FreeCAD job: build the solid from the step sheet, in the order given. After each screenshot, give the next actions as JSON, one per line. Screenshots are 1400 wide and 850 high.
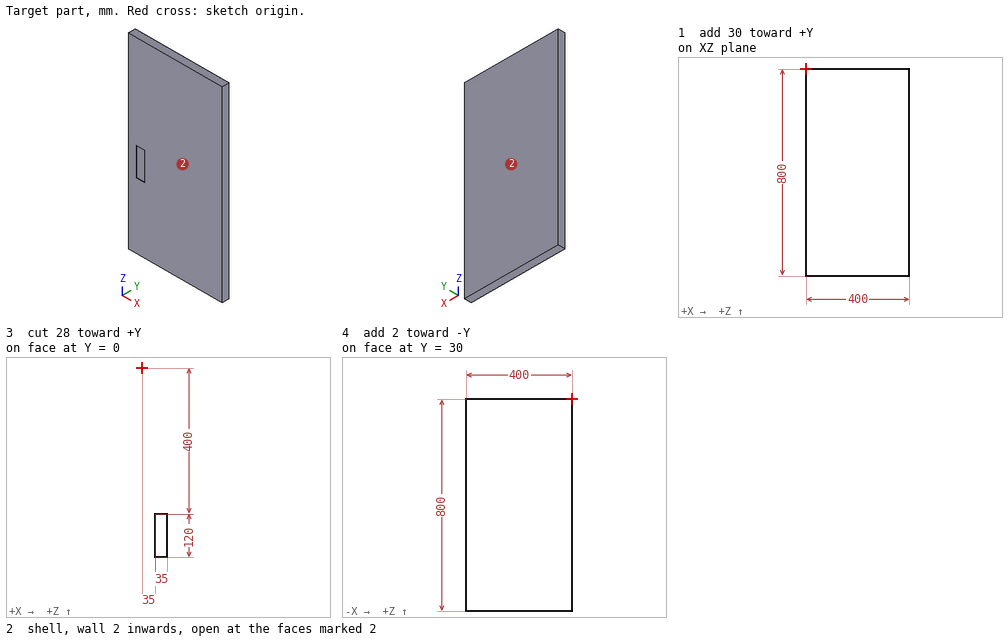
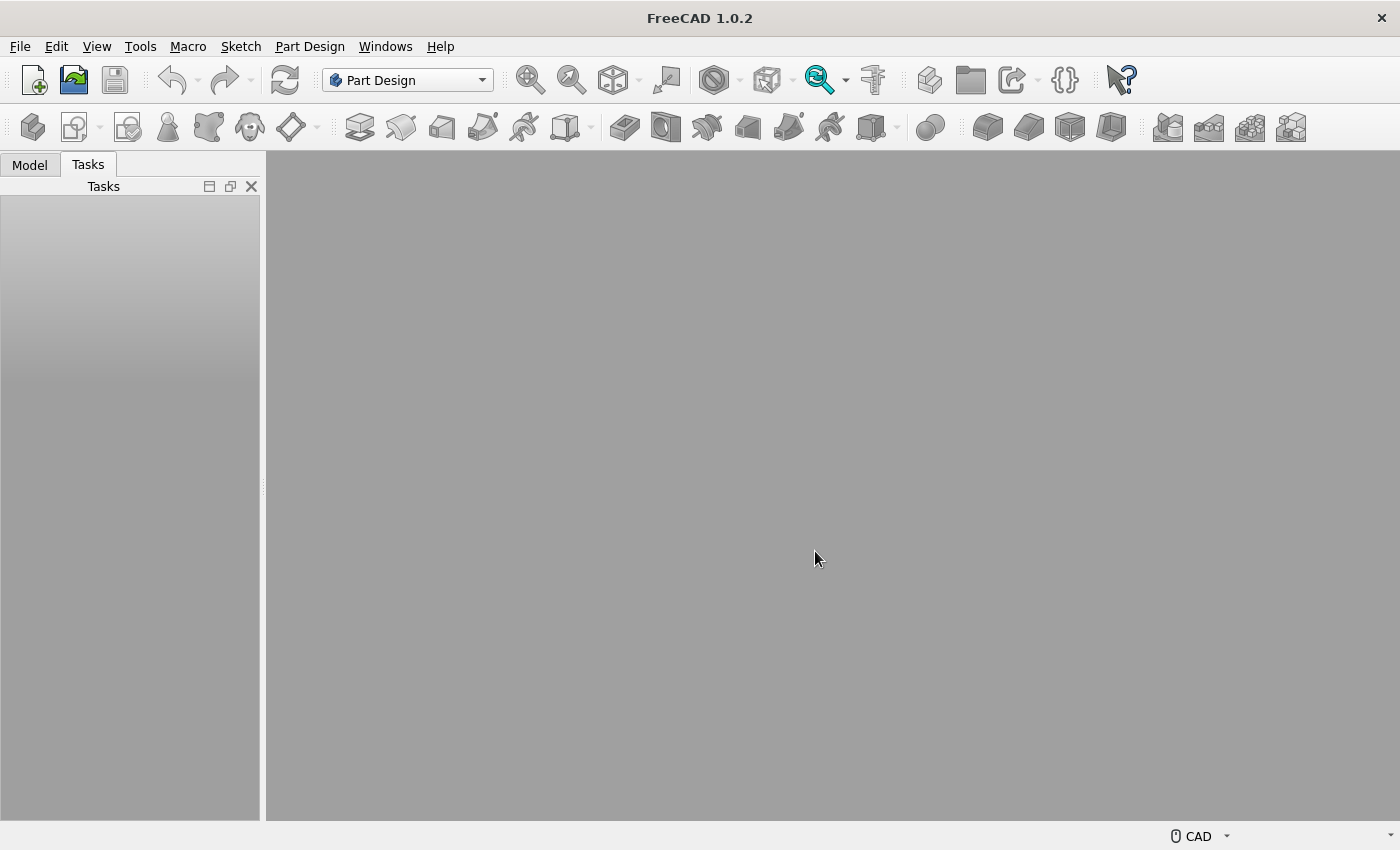
{"action": "left_click", "coordinate": [33, 80]}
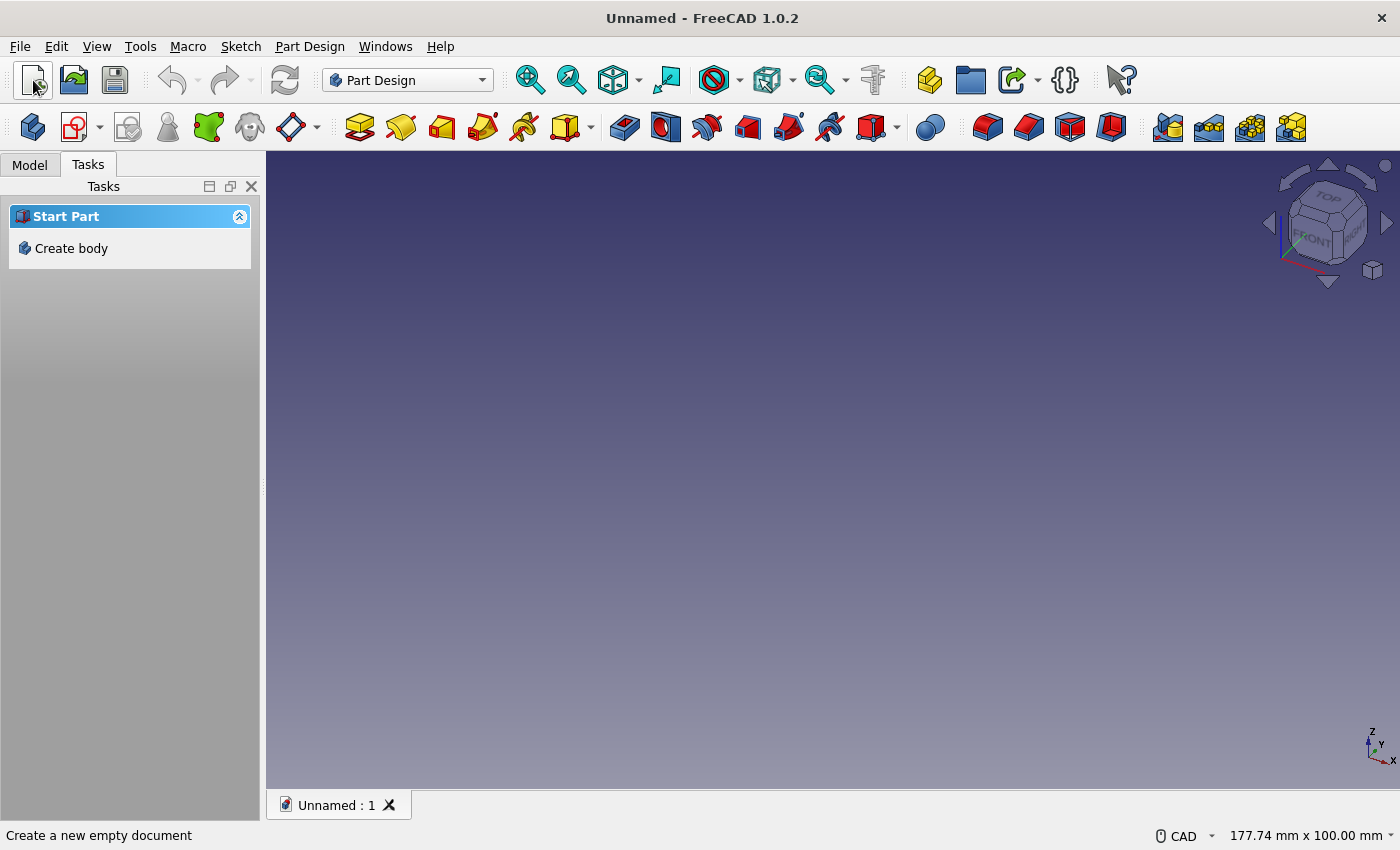
{"action": "left_click", "coordinate": [74, 128]}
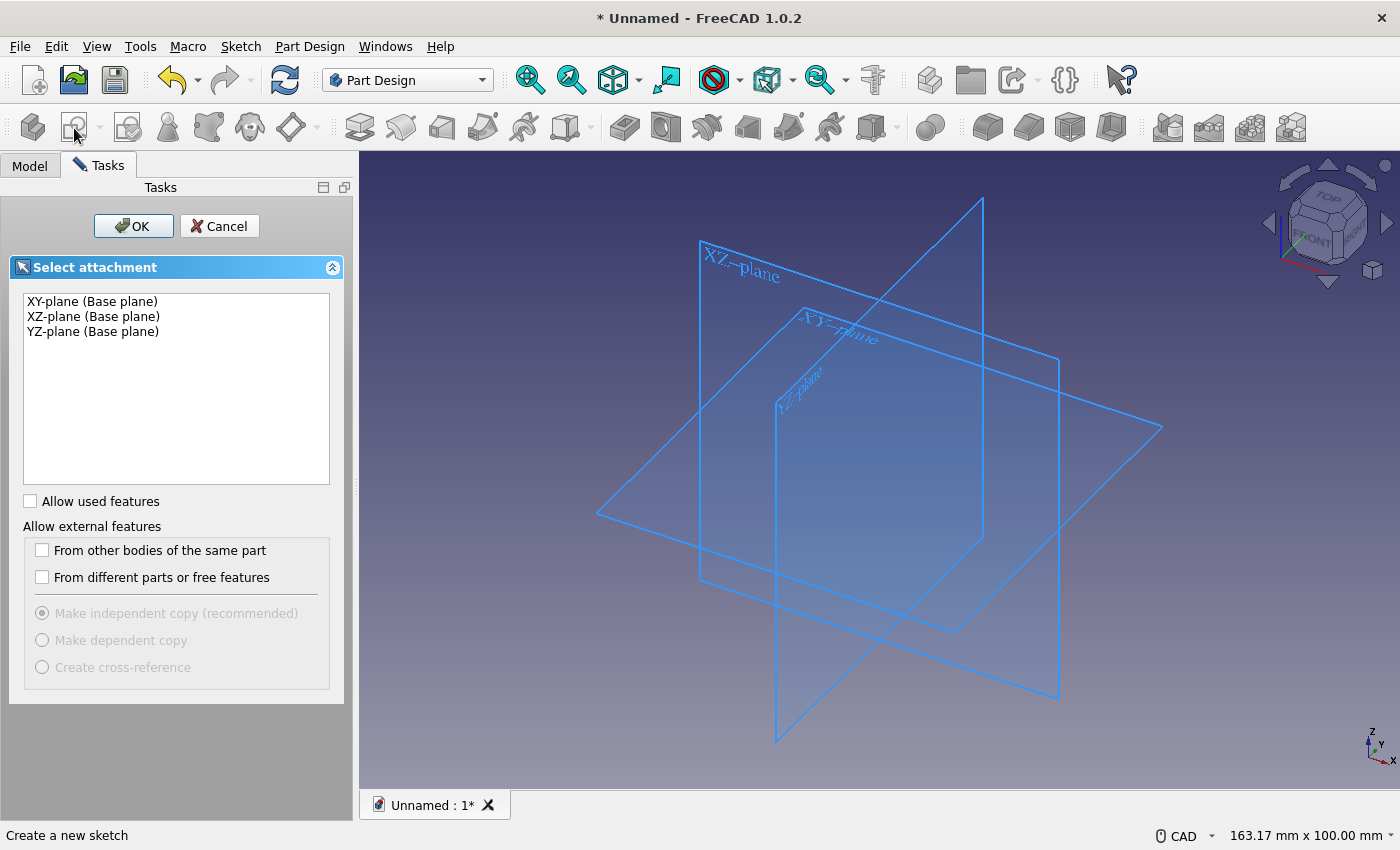
{"action": "left_click", "coordinate": [84, 316]}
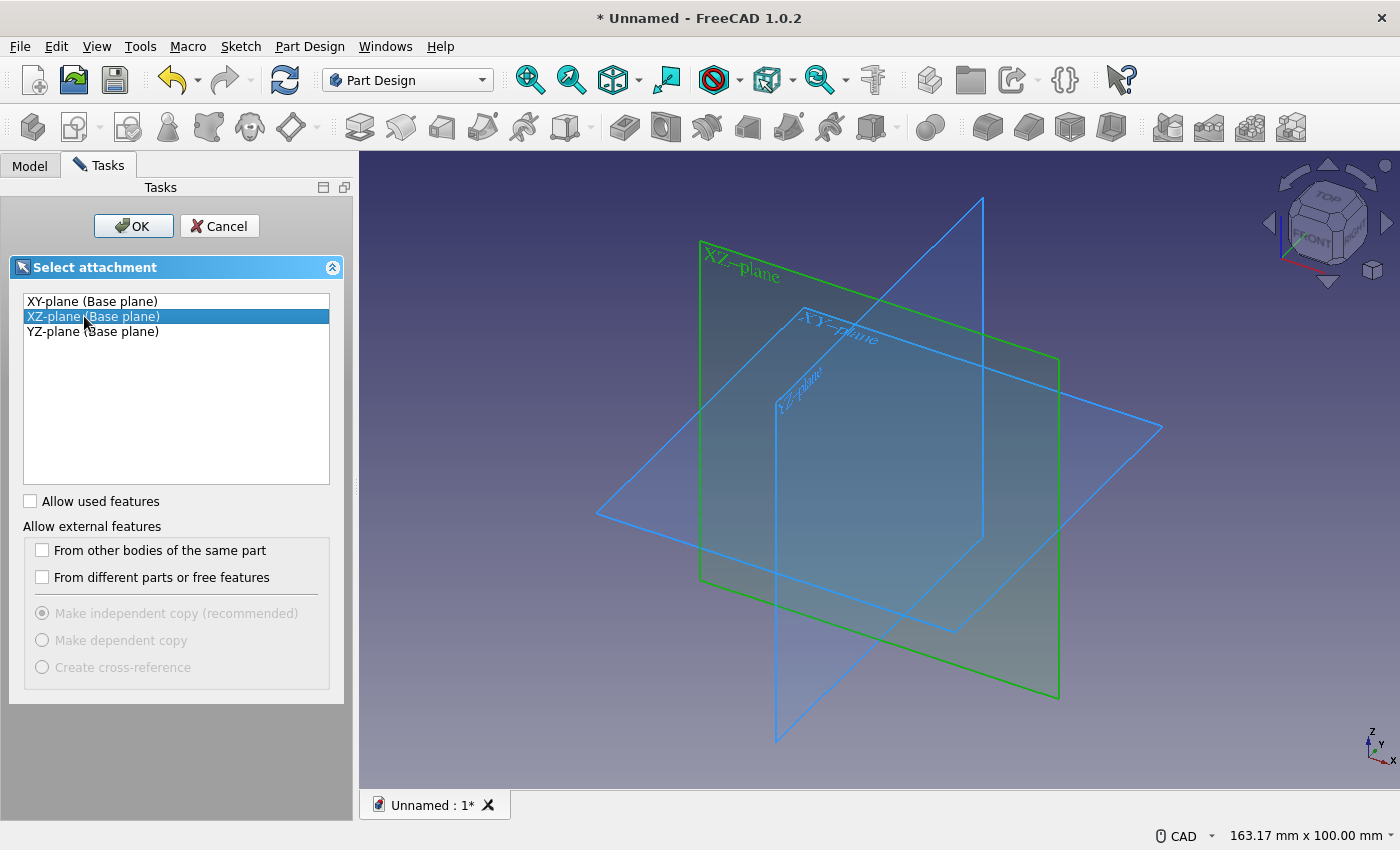
{"action": "left_click", "coordinate": [134, 226]}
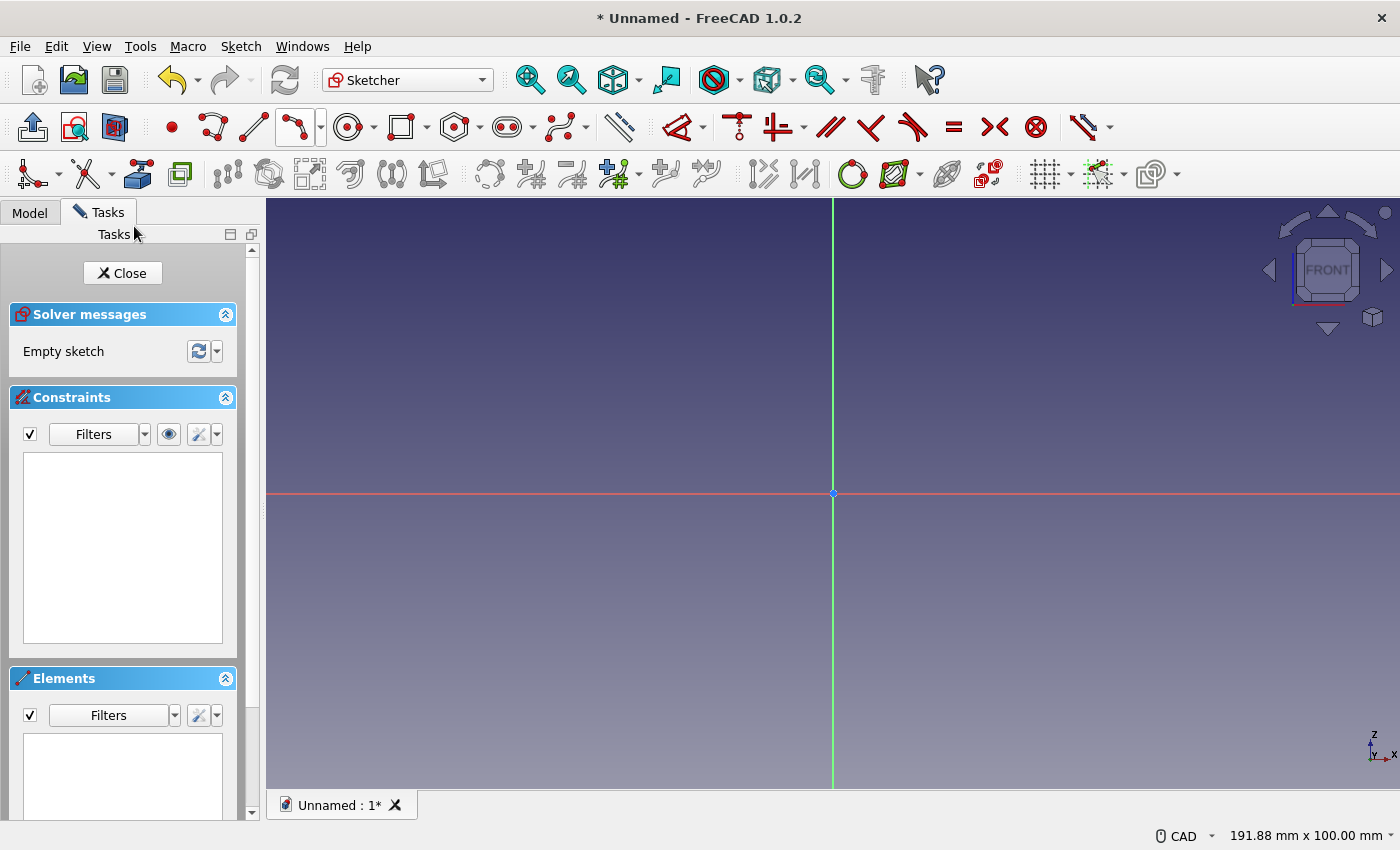
{"action": "scroll", "coordinate": [664, 304], "scroll_direction": "down", "scroll_amount": 13}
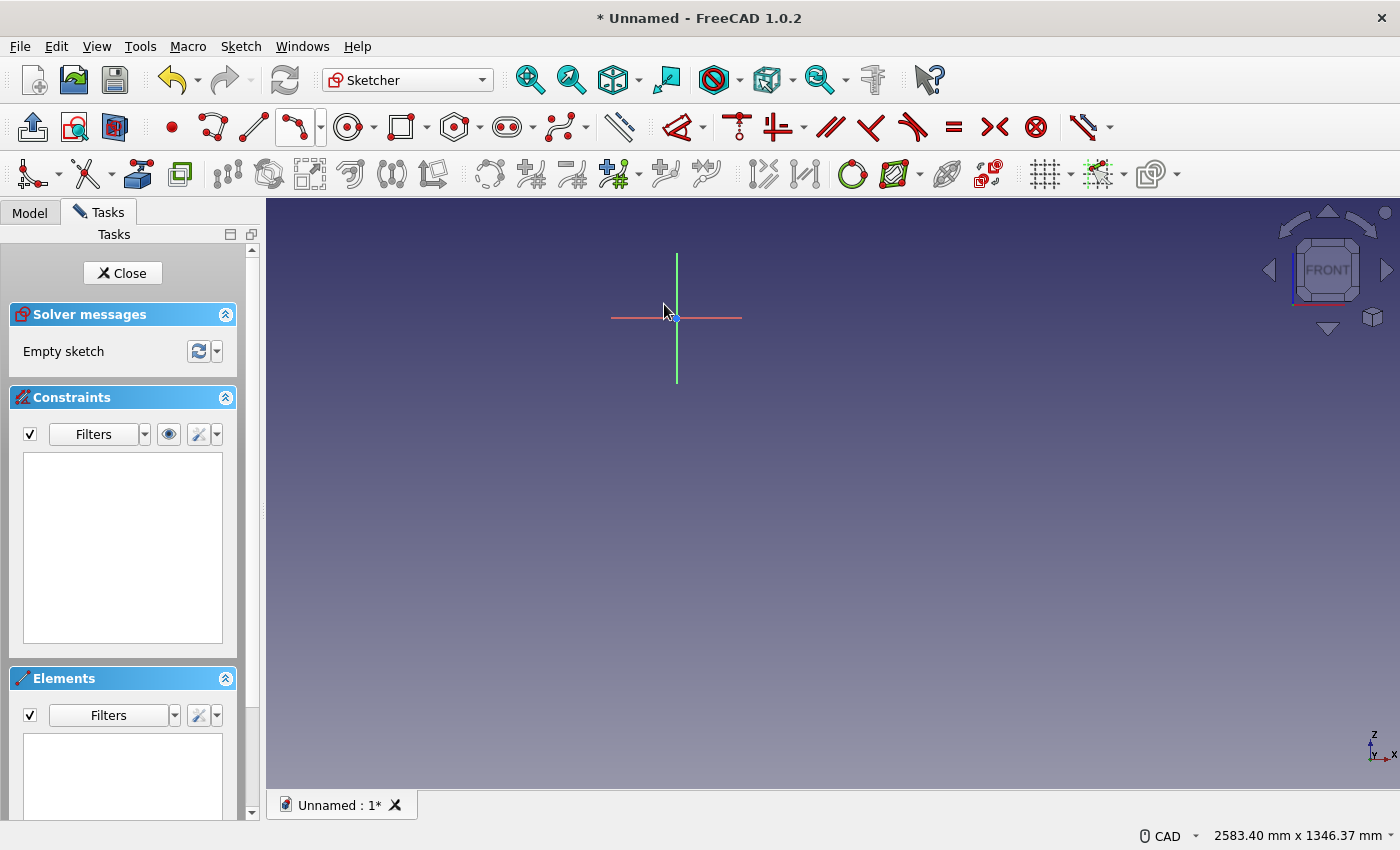
{"action": "key", "text": "g r"}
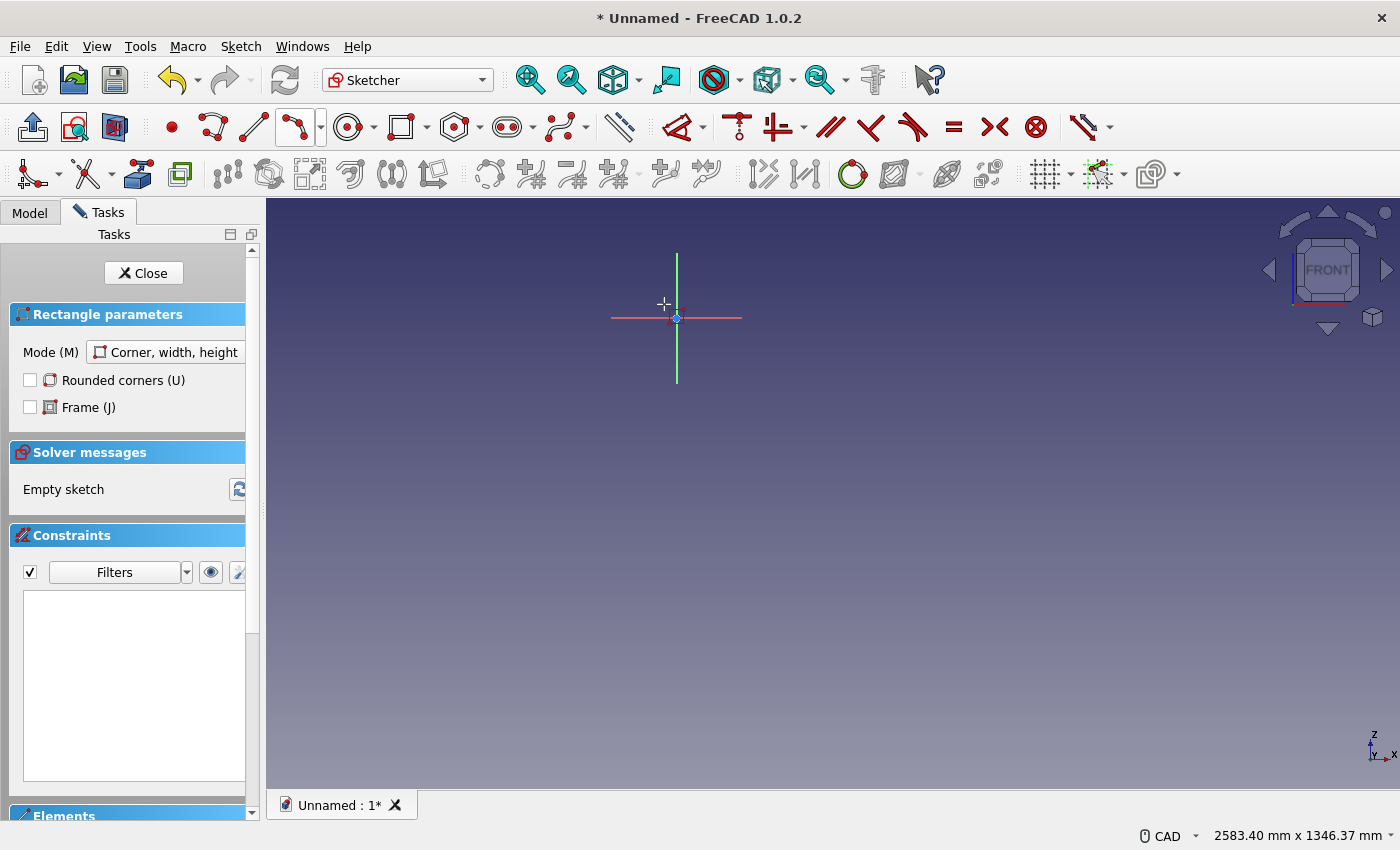
{"action": "left_click", "coordinate": [677, 318]}
{"action": "left_click", "coordinate": [852, 669]}
{"action": "key", "text": "Escape"}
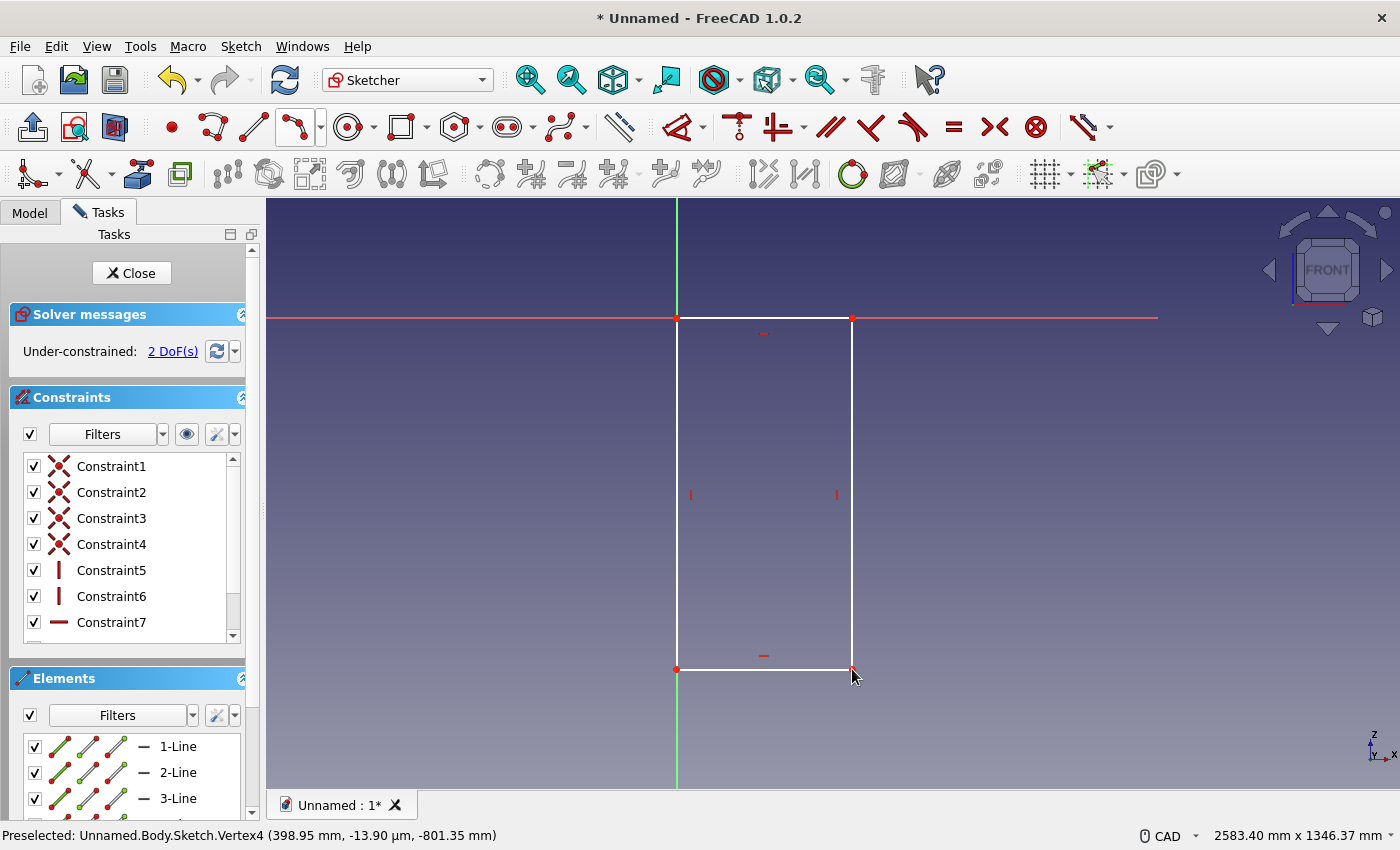
{"action": "left_click", "coordinate": [676, 128]}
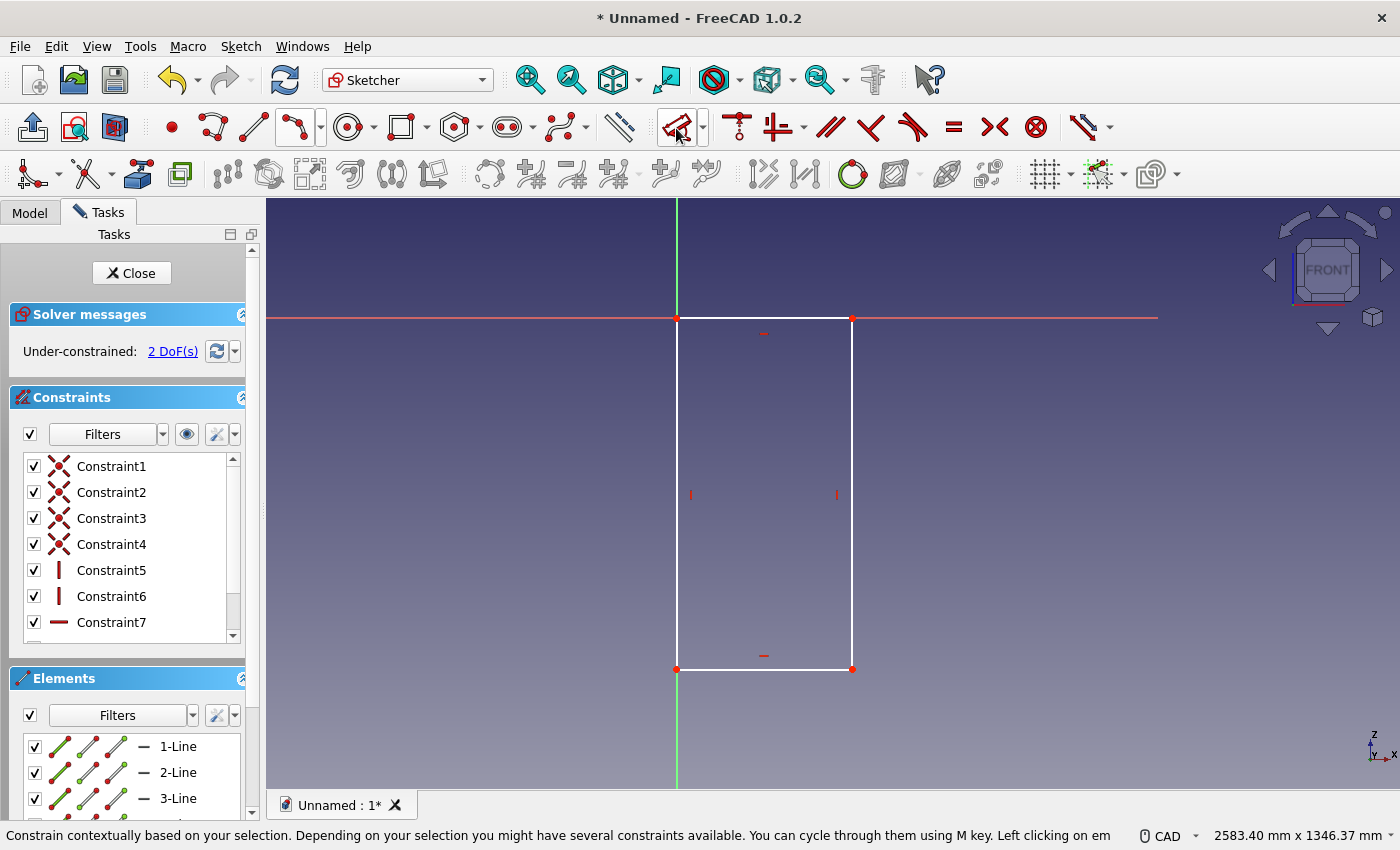
{"action": "left_click", "coordinate": [677, 424]}
{"action": "left_click", "coordinate": [643, 494]}